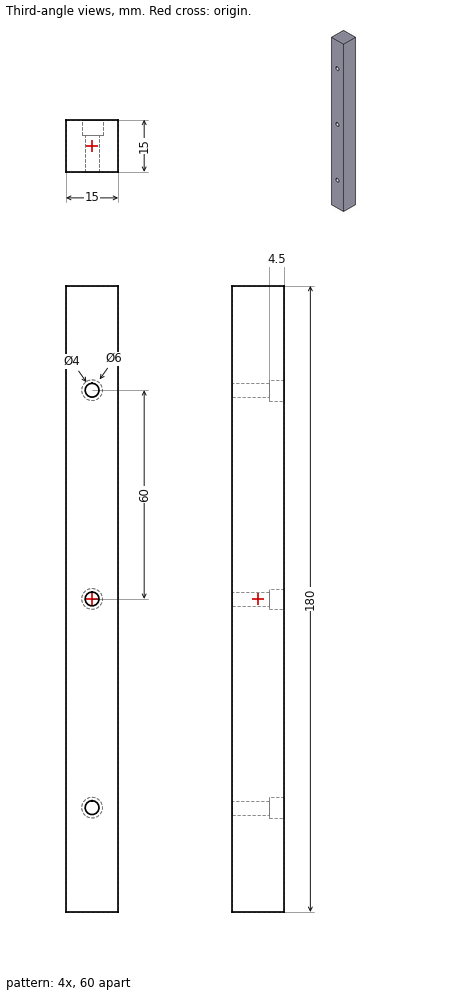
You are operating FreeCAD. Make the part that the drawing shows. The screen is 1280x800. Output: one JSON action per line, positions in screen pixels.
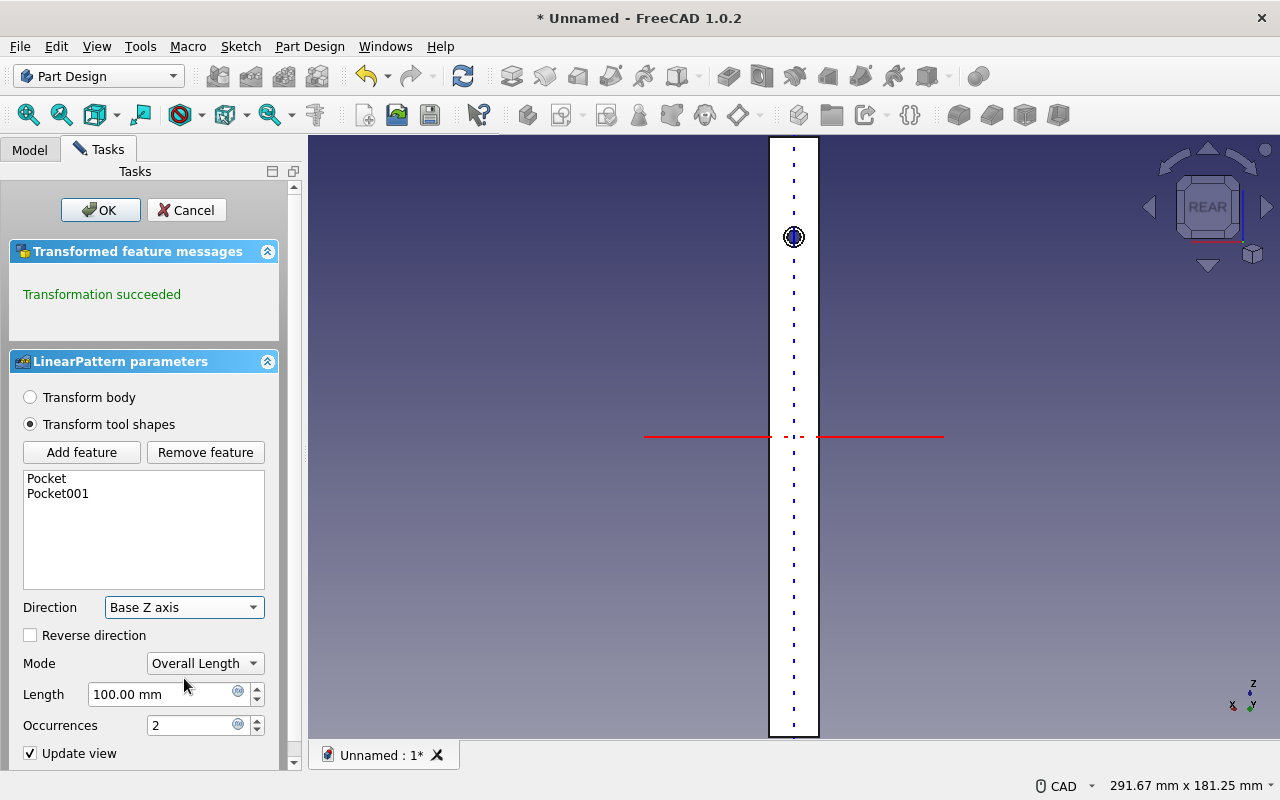
{"action": "left_click", "coordinate": [206, 664]}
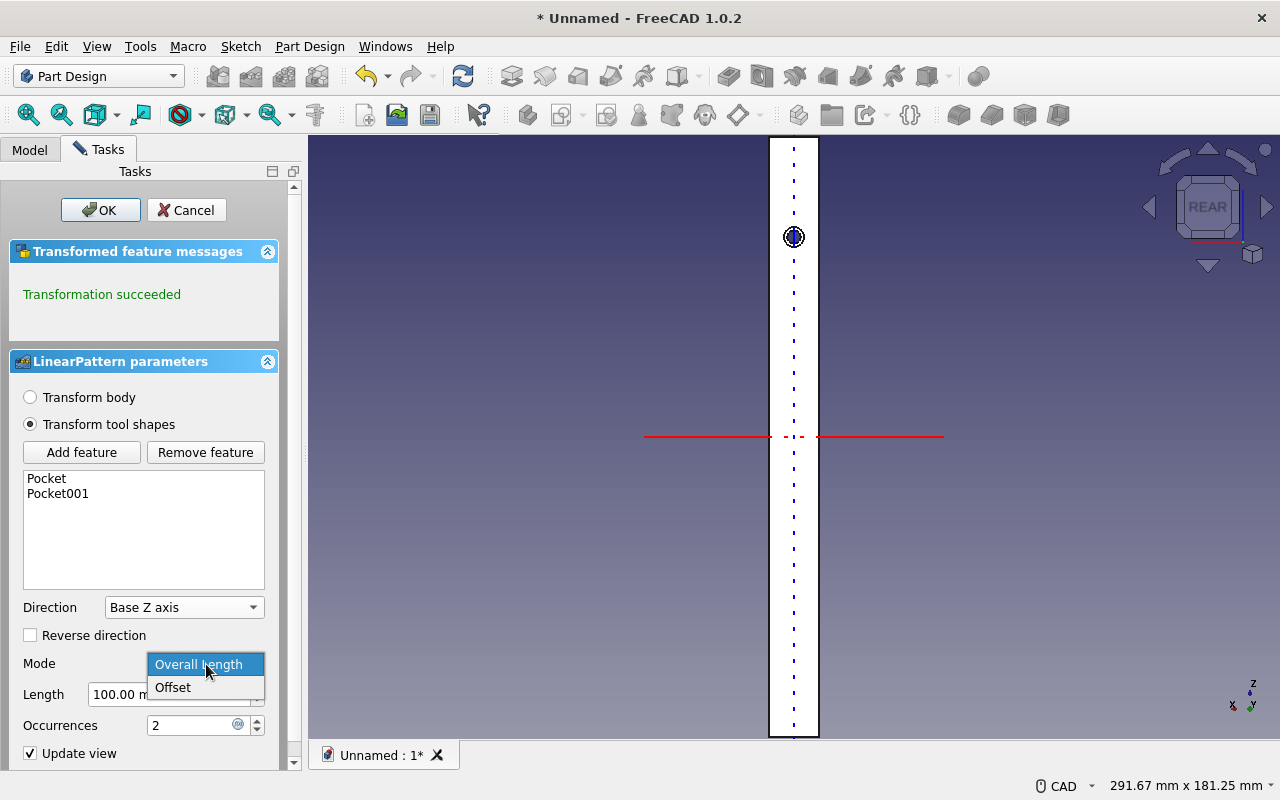
{"action": "left_click", "coordinate": [204, 688]}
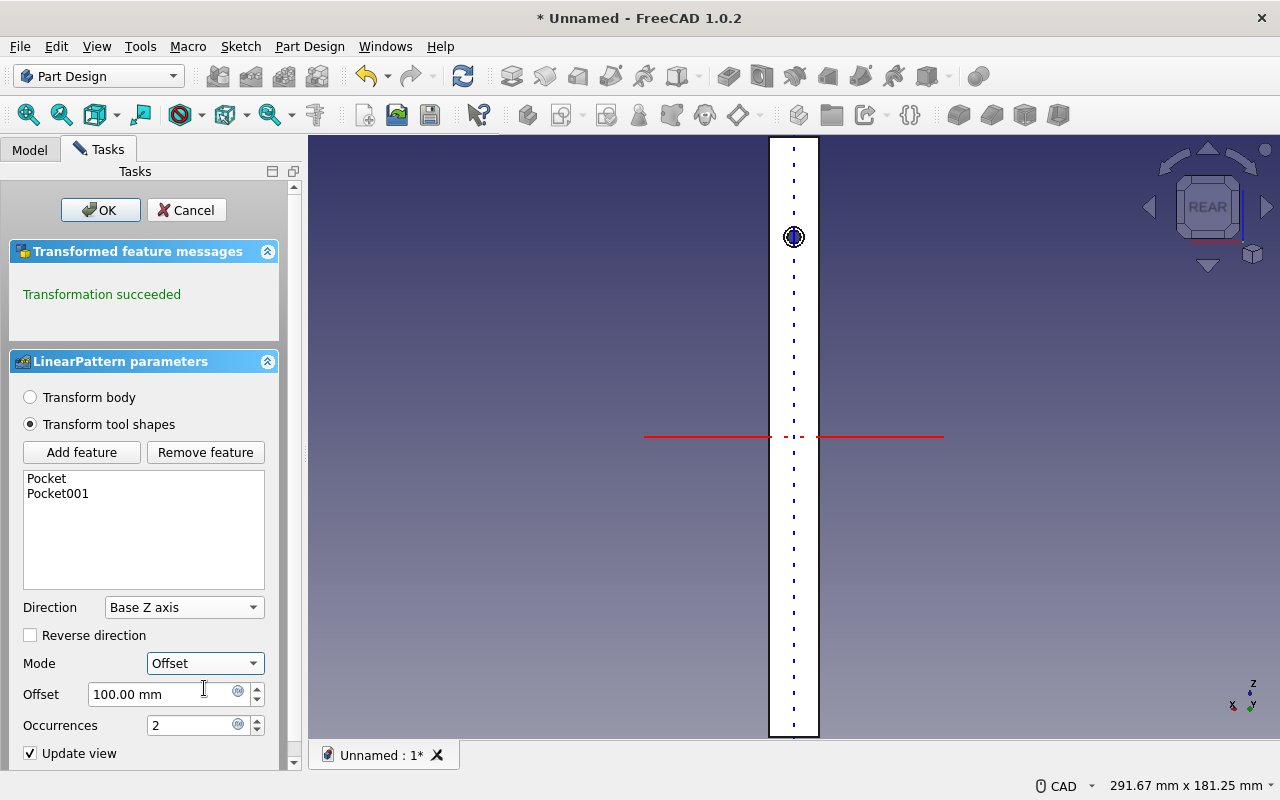
{"action": "triple_click", "coordinate": [170, 694]}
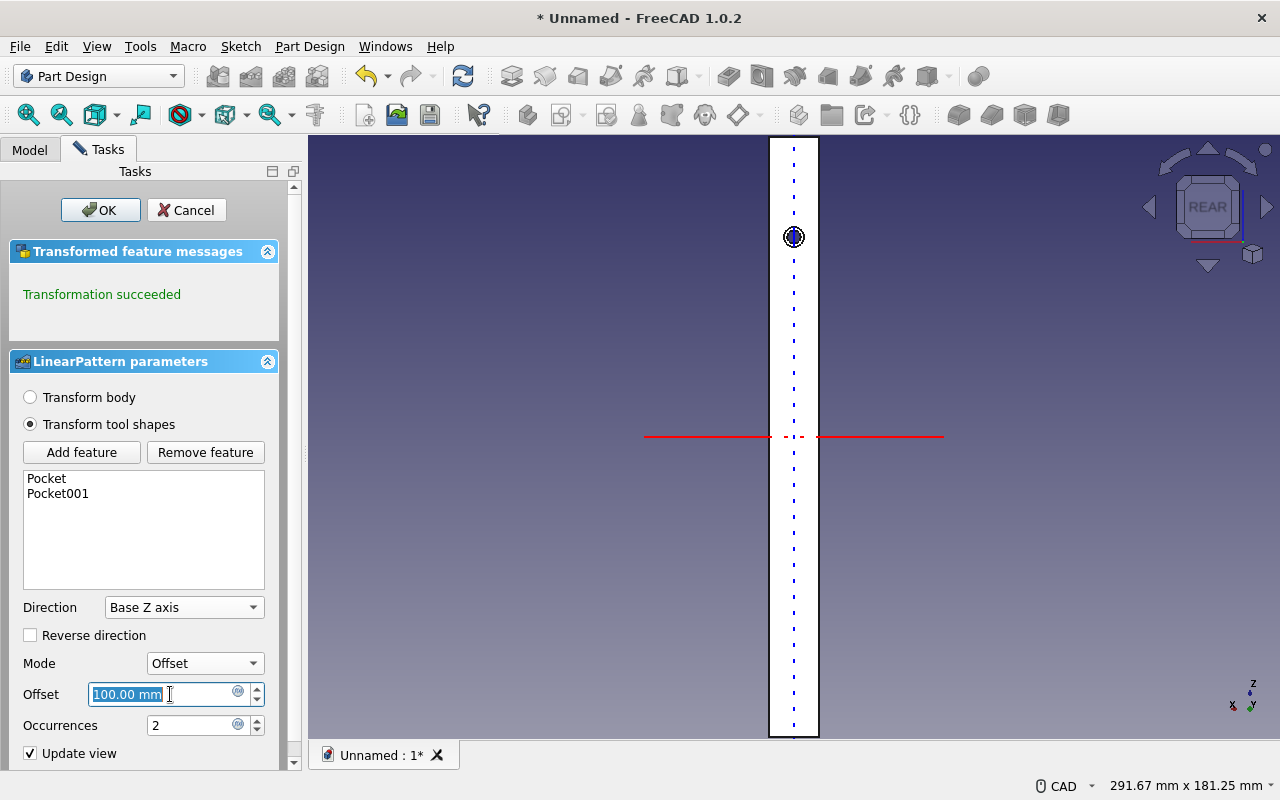
{"action": "type", "text": "60"}
{"action": "key", "text": "Tab"}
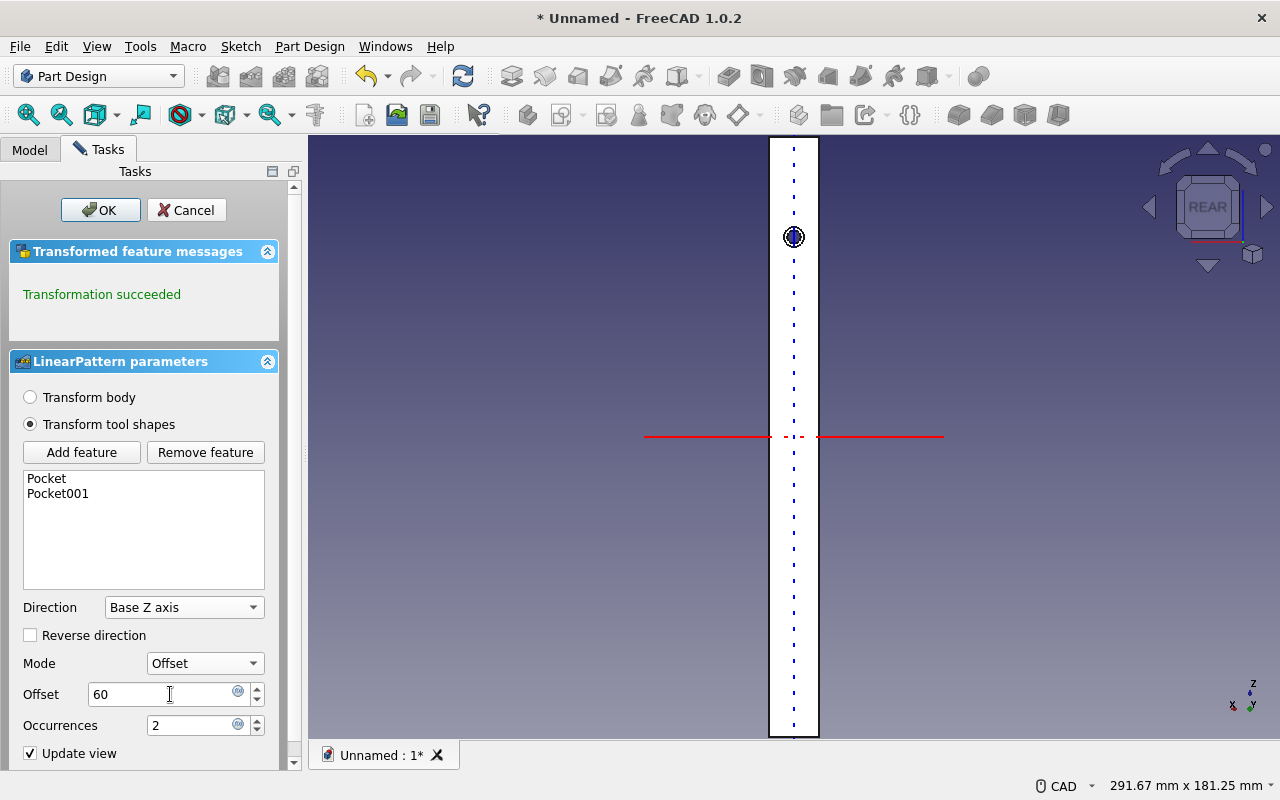
{"action": "triple_click", "coordinate": [199, 726]}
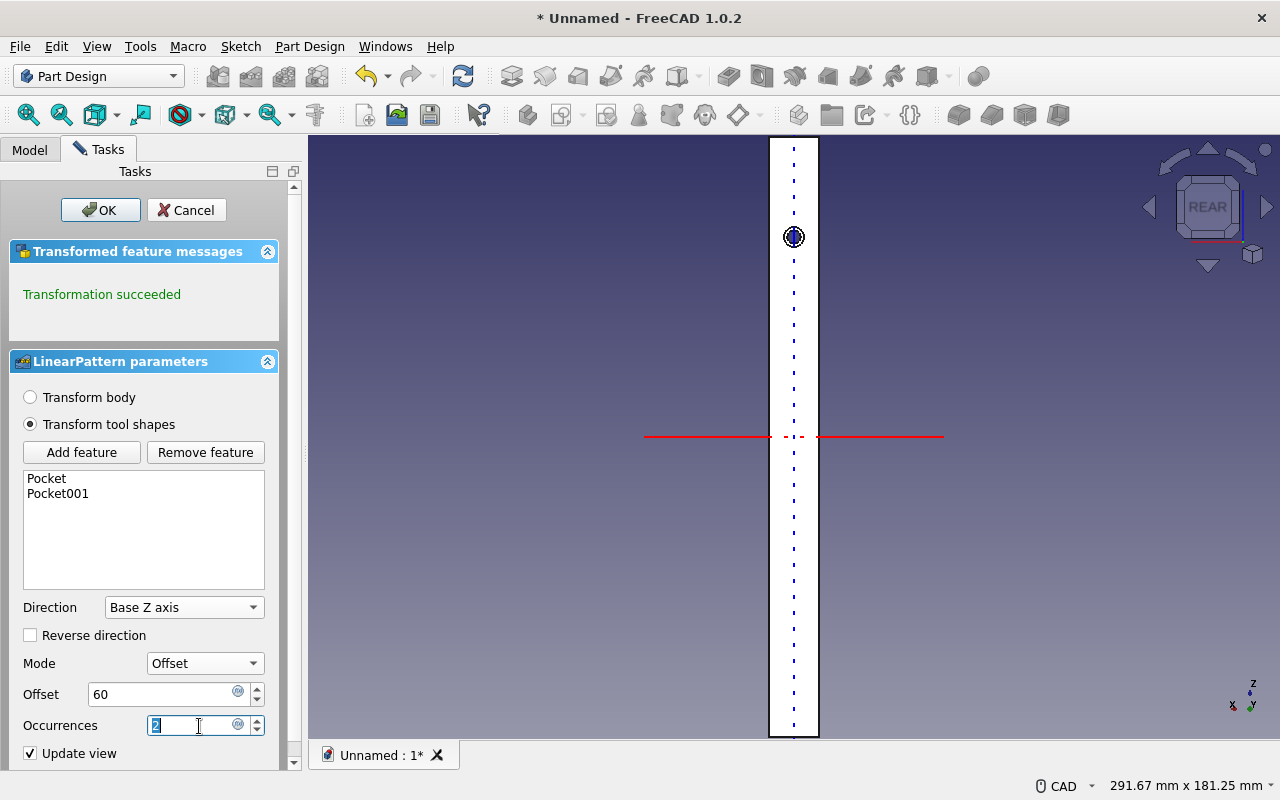
{"action": "type", "text": "4"}
{"action": "key", "text": "Tab"}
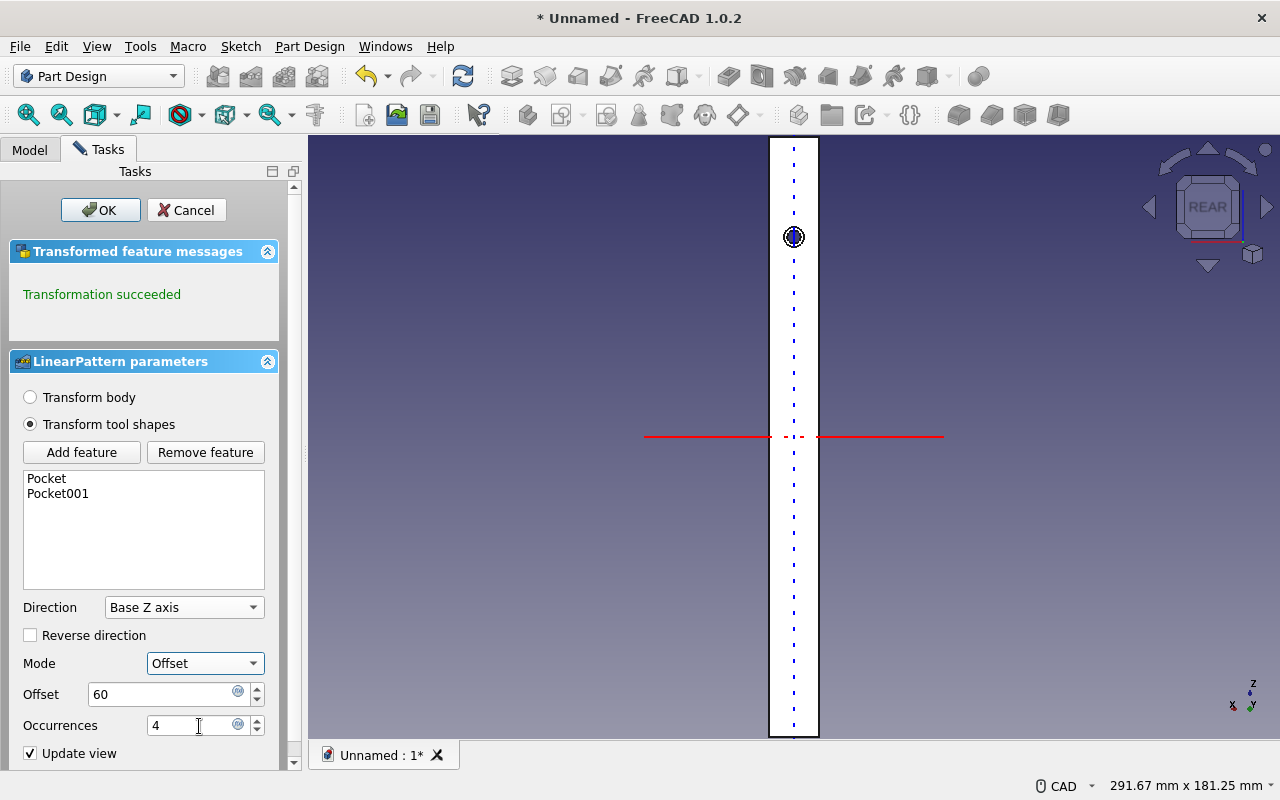
{"action": "left_click", "coordinate": [31, 635]}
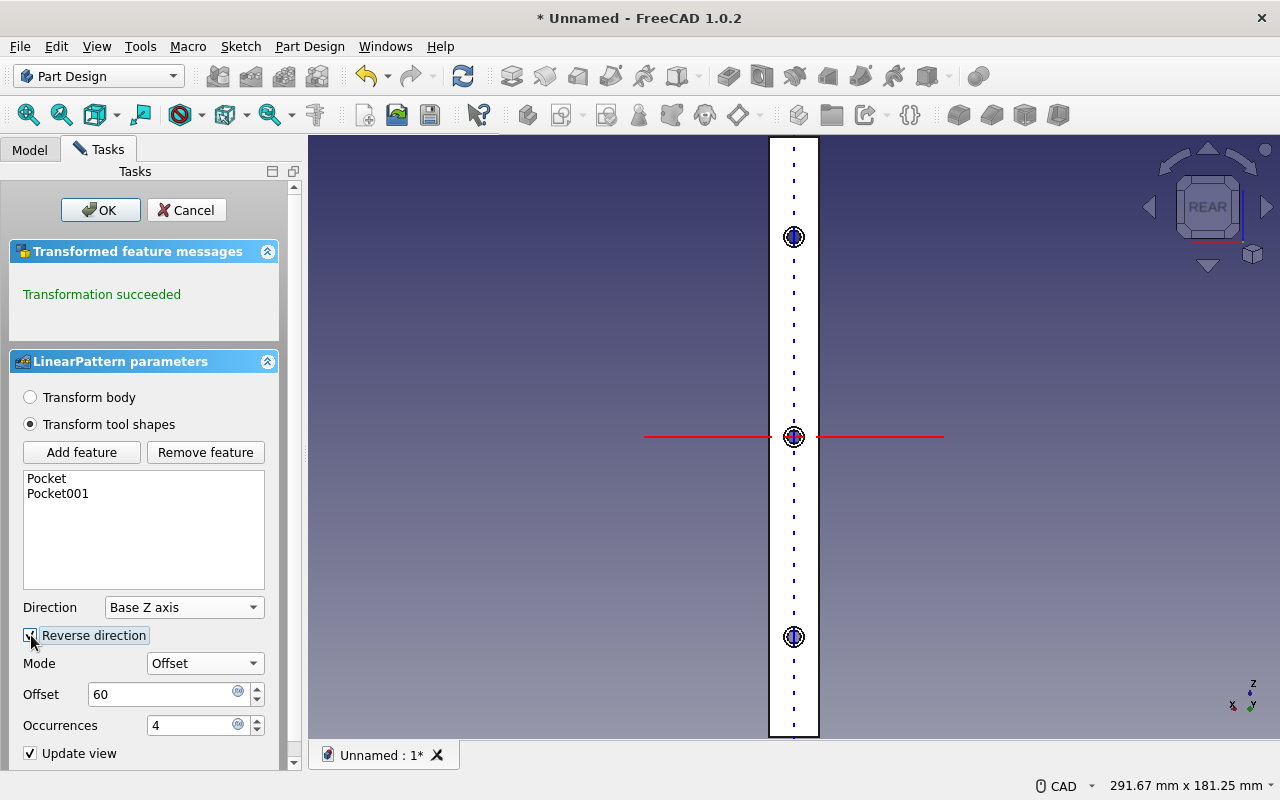
{"action": "left_click", "coordinate": [101, 210]}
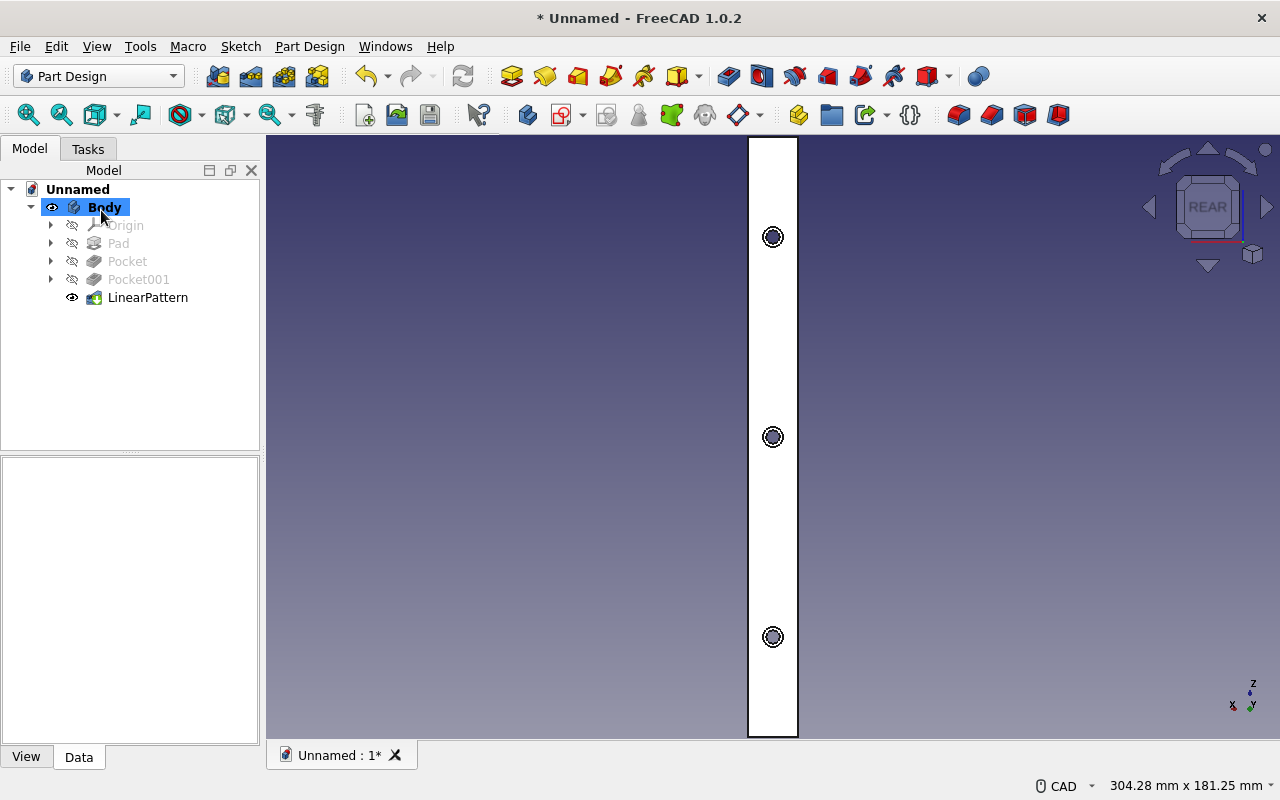
{"action": "key", "text": "0"}